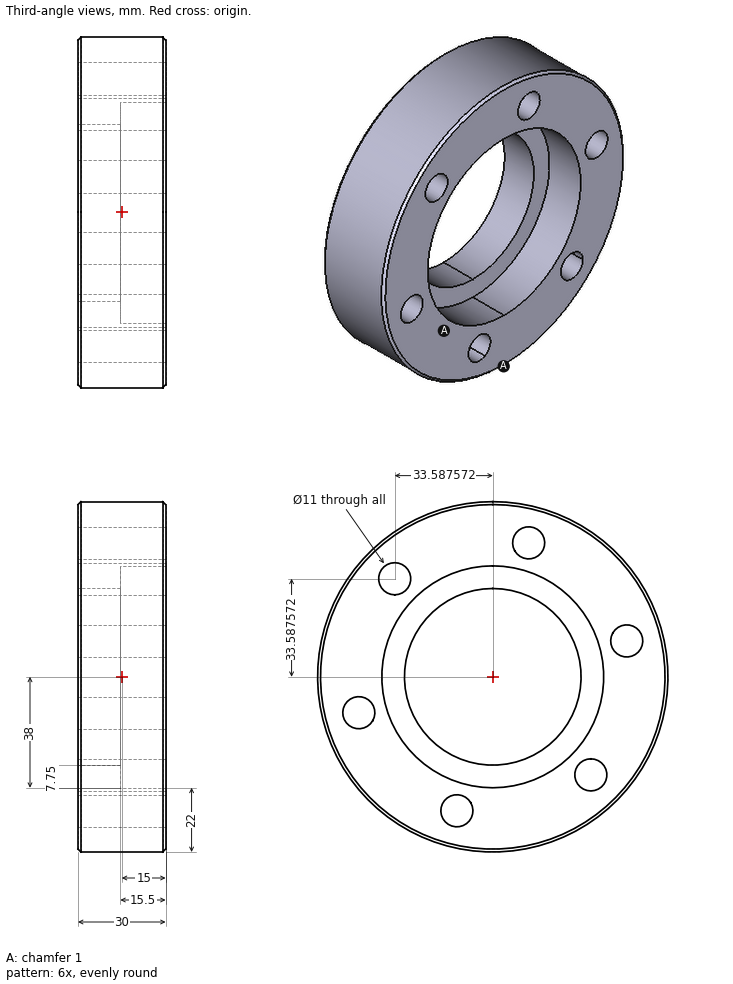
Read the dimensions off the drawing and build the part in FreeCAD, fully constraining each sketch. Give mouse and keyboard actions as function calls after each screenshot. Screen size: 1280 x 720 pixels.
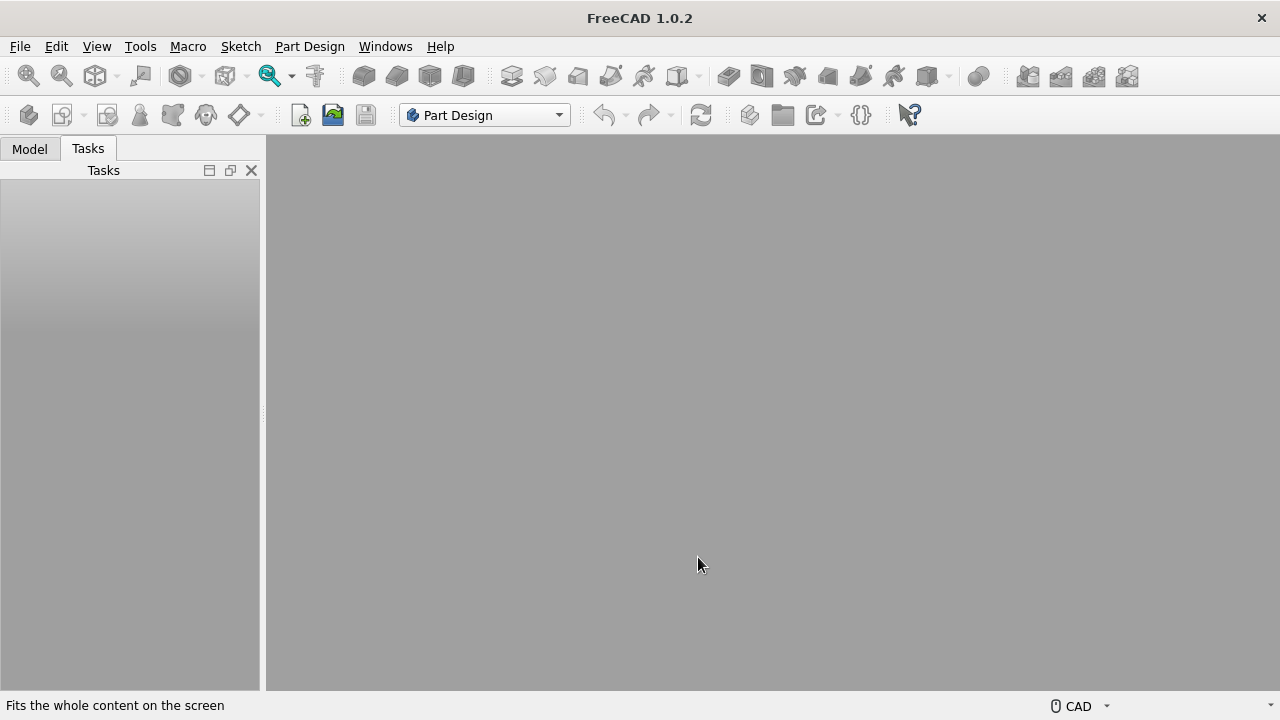
key(ctrl+n)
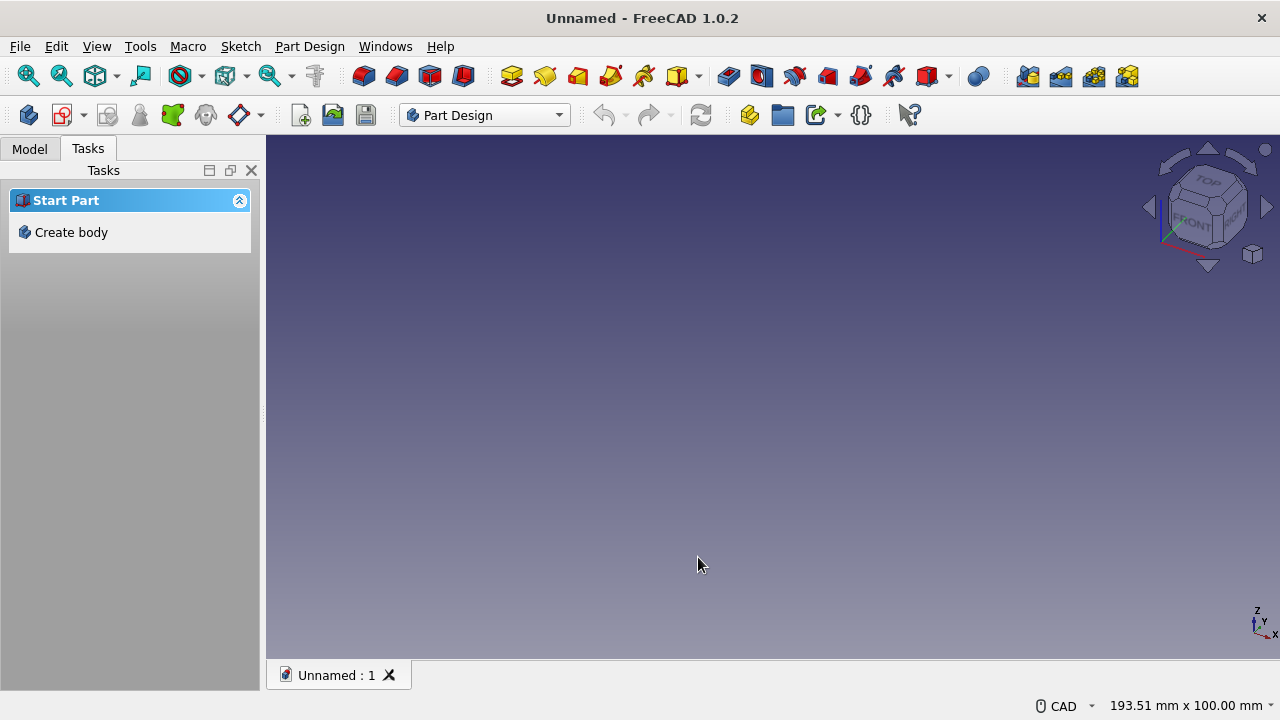
click(62, 116)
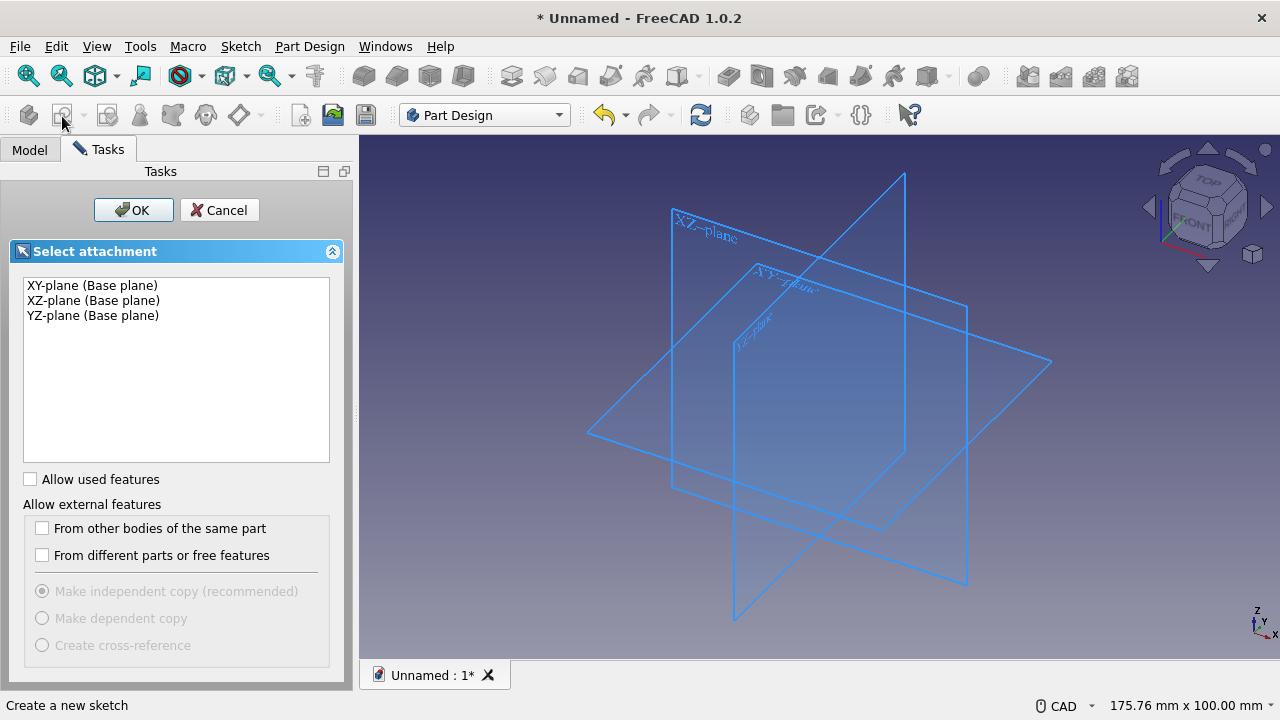
click(84, 300)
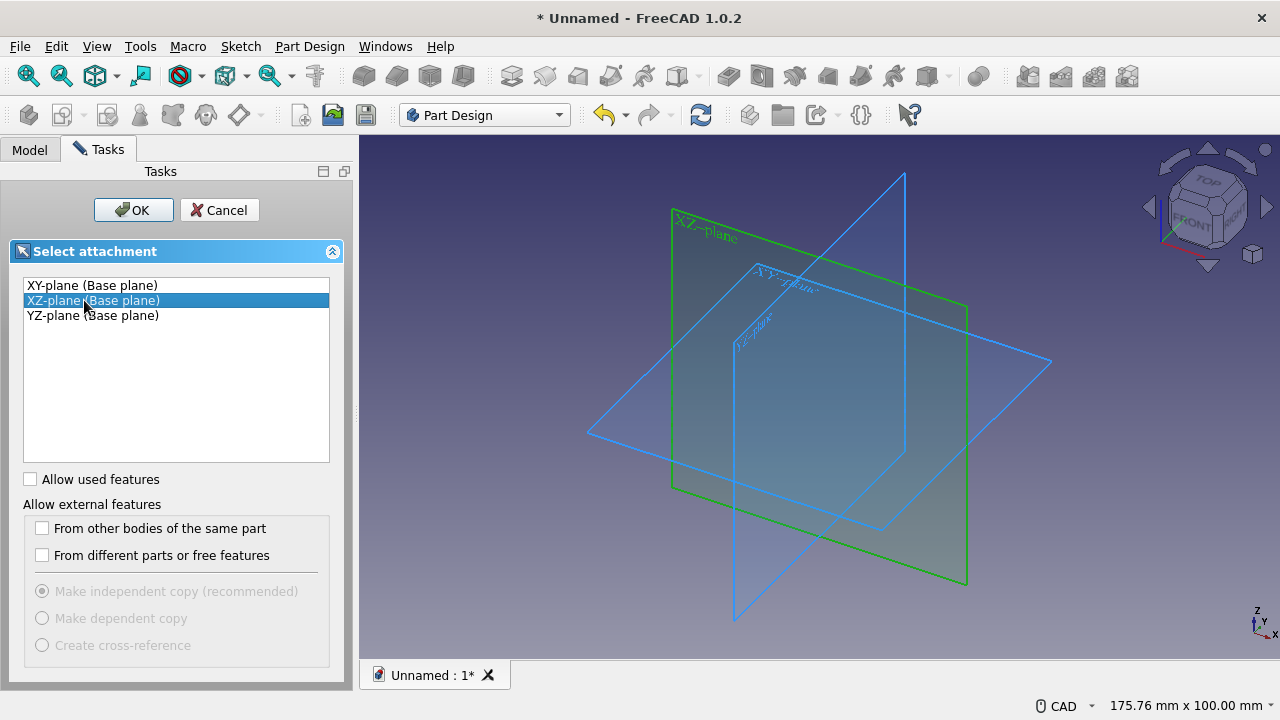
click(134, 210)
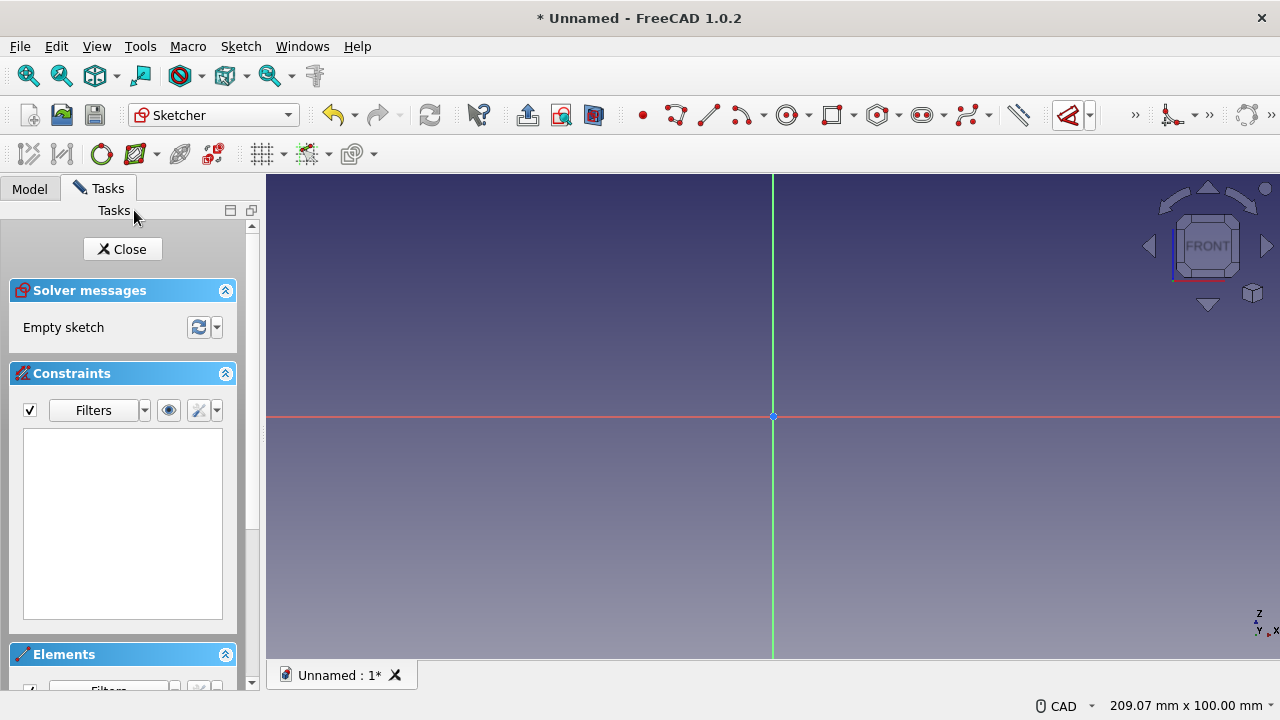
scroll(565, 202, down, 2)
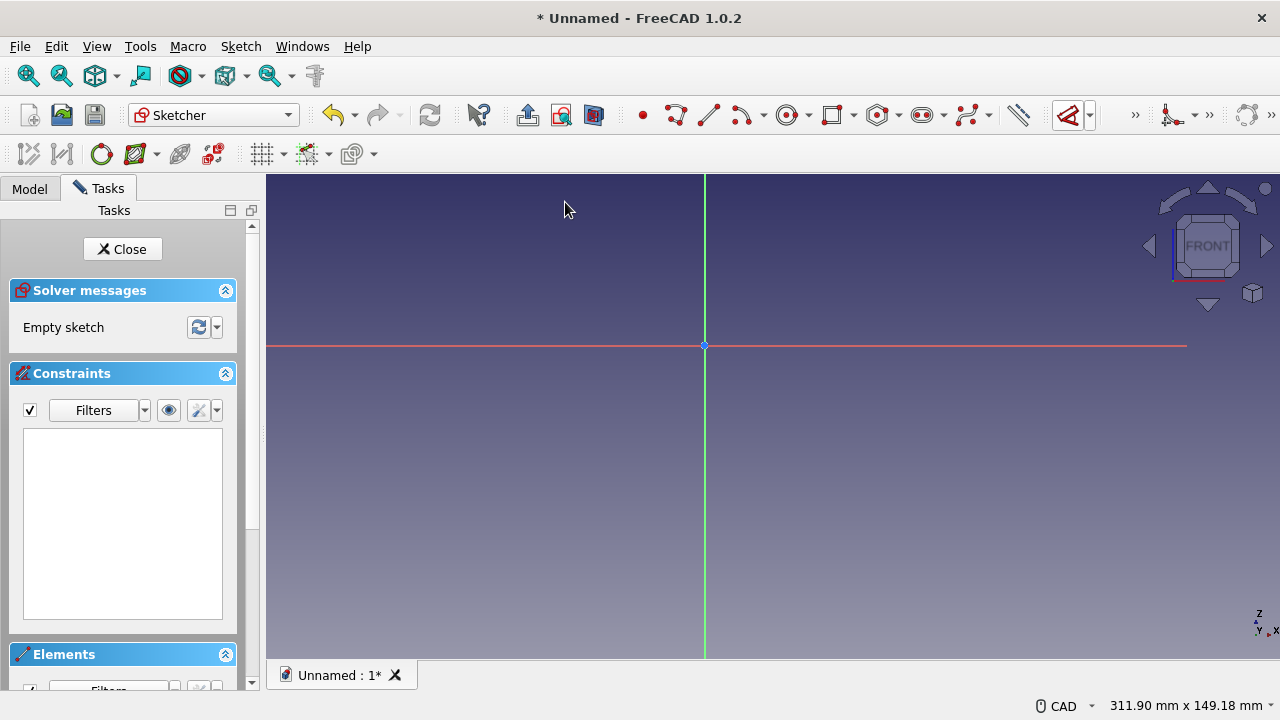
scroll(705, 498, up, 2)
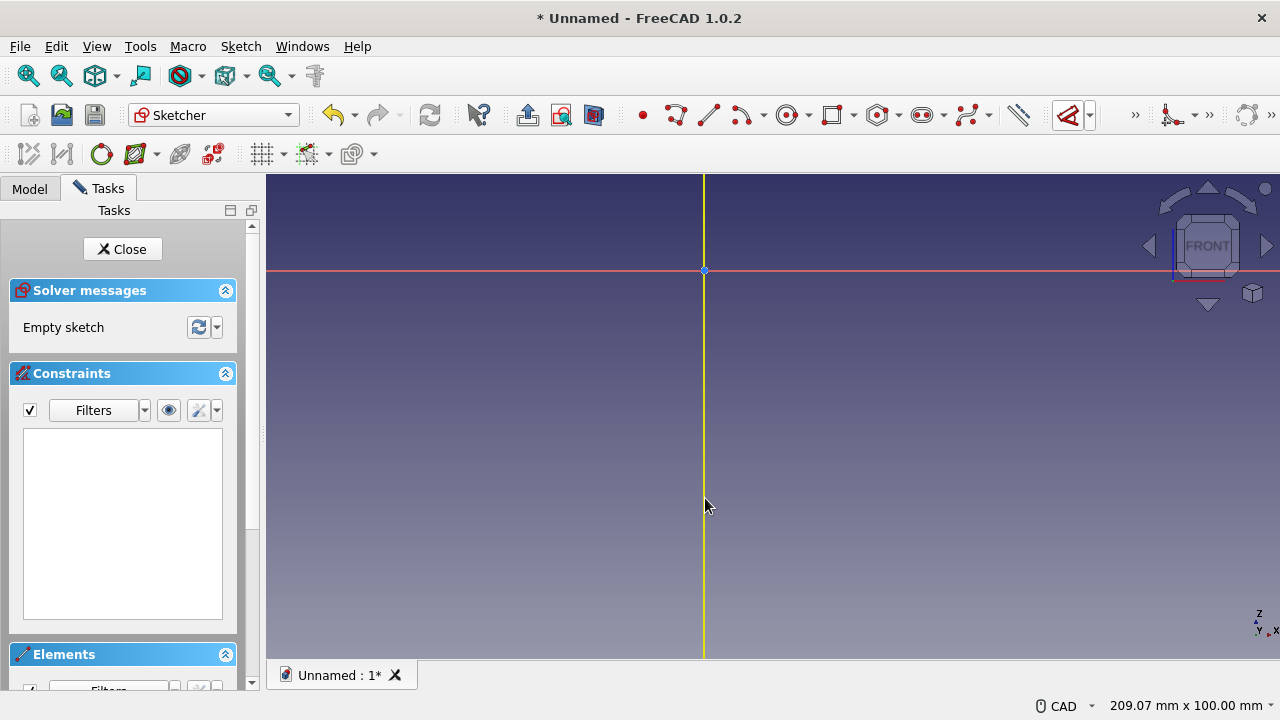
key(g)
key(m)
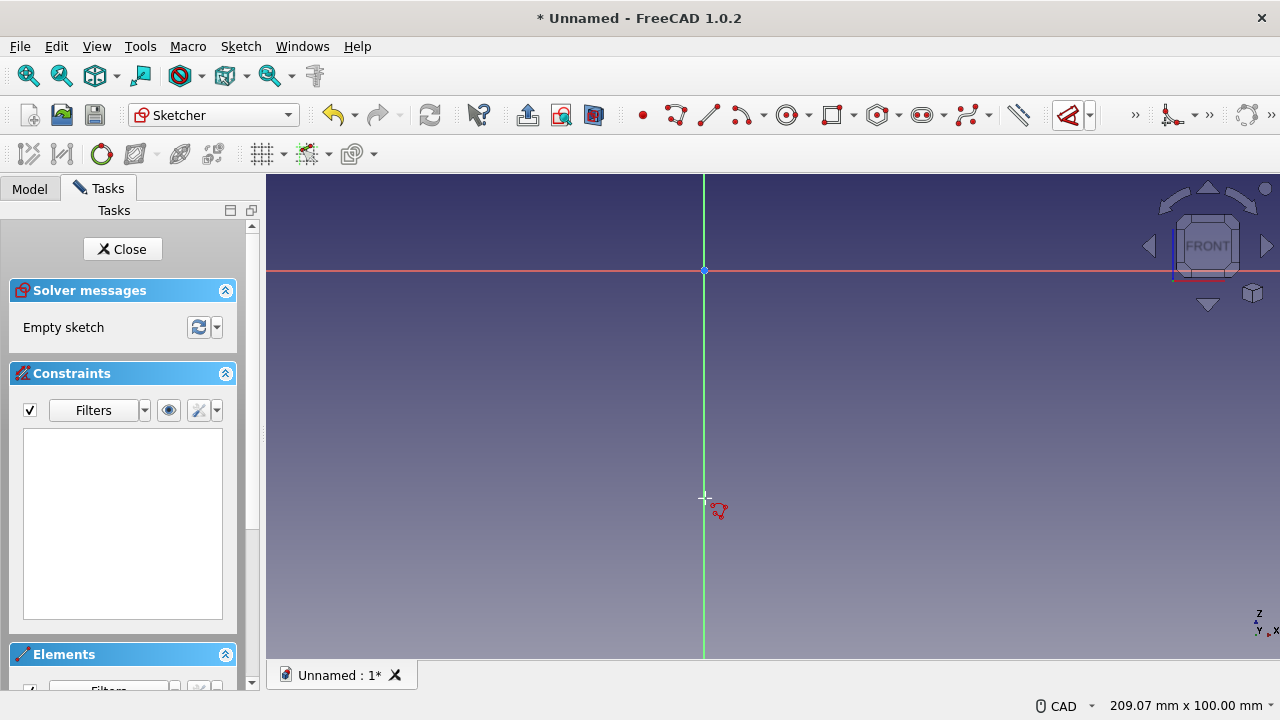
scroll(702, 417, up, 10)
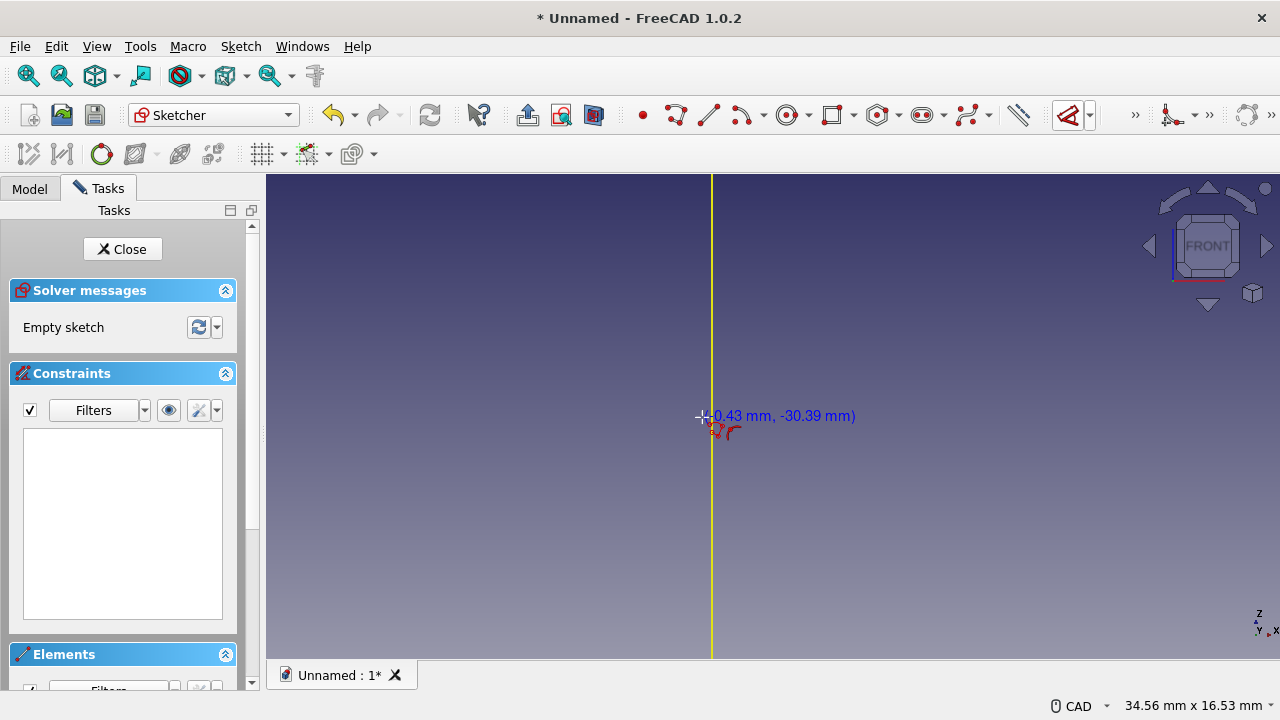
click(697, 416)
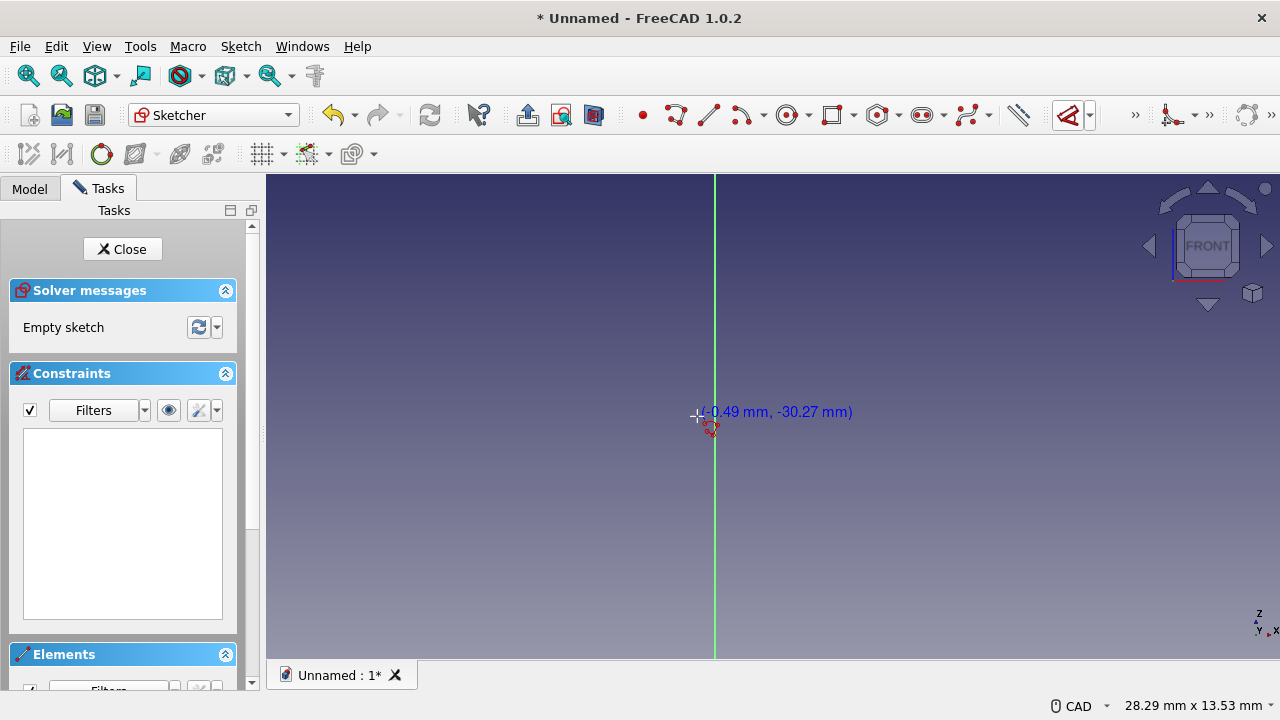
scroll(703, 418, down, 10)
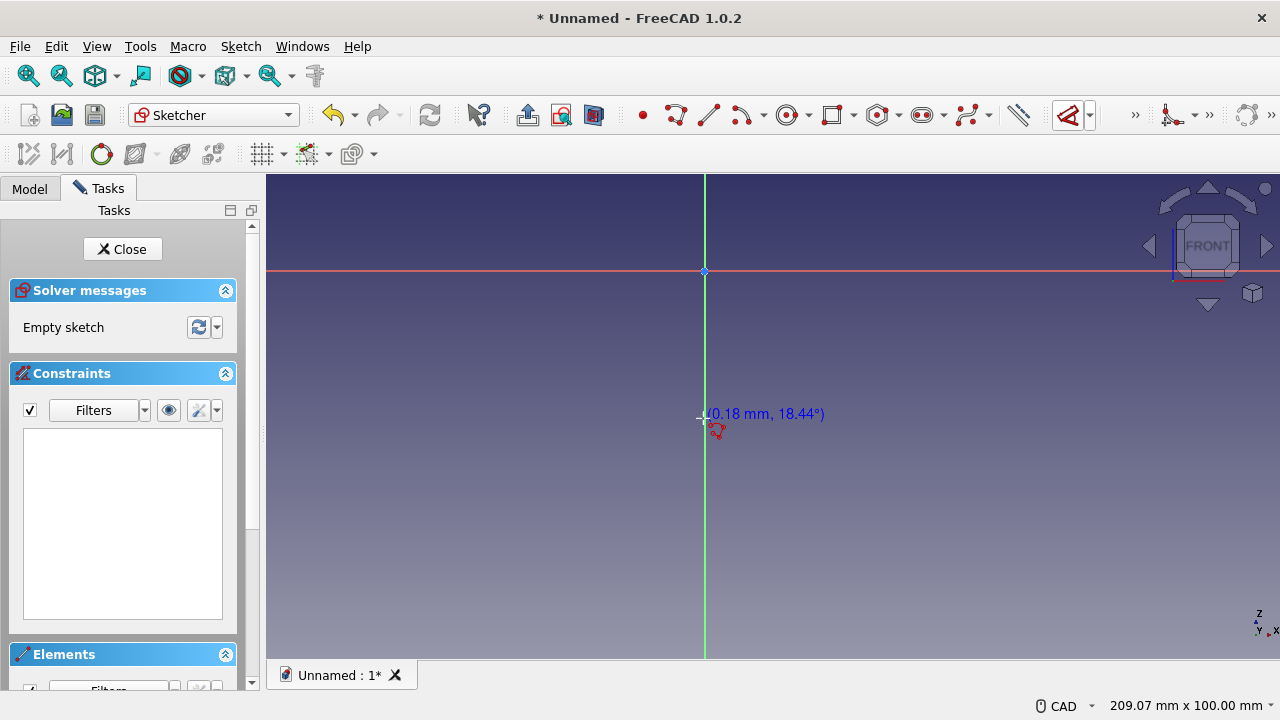
scroll(703, 456, up, 10)